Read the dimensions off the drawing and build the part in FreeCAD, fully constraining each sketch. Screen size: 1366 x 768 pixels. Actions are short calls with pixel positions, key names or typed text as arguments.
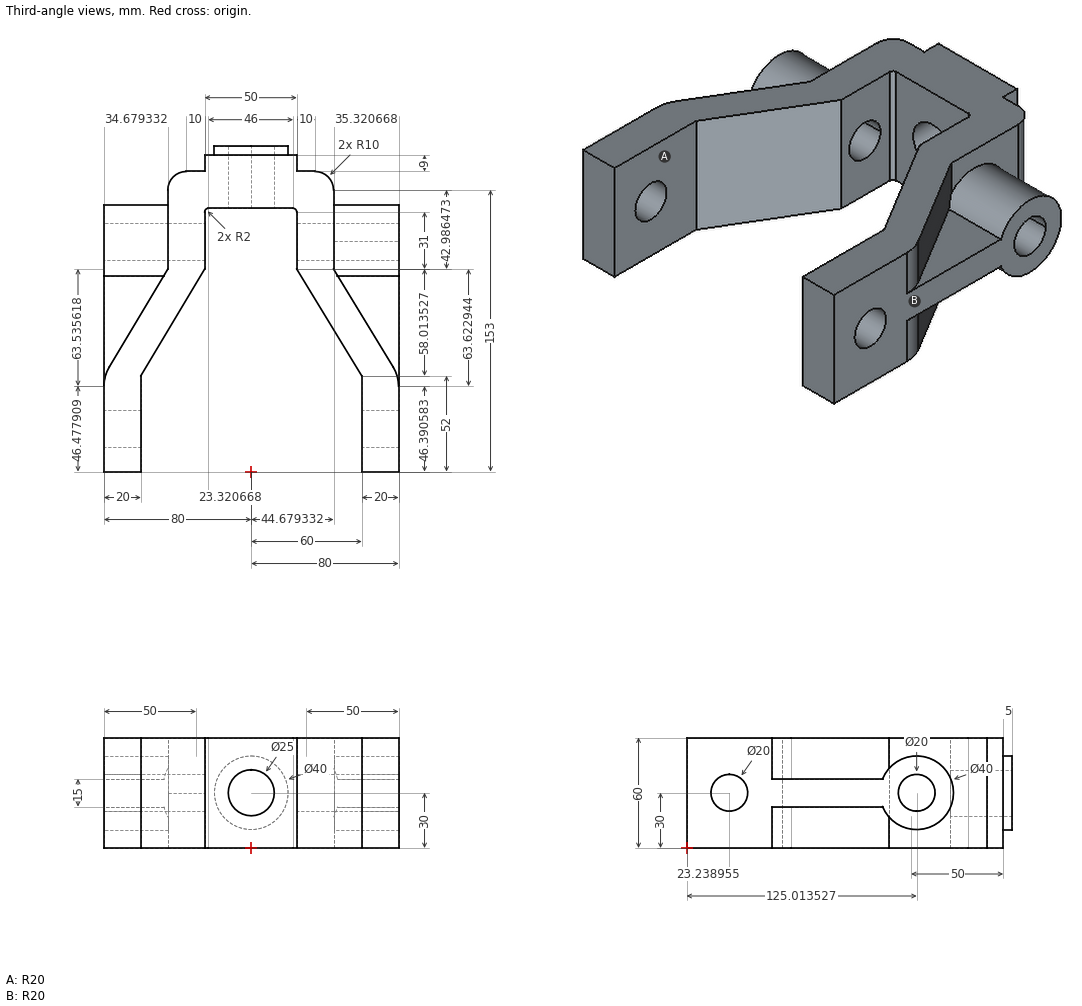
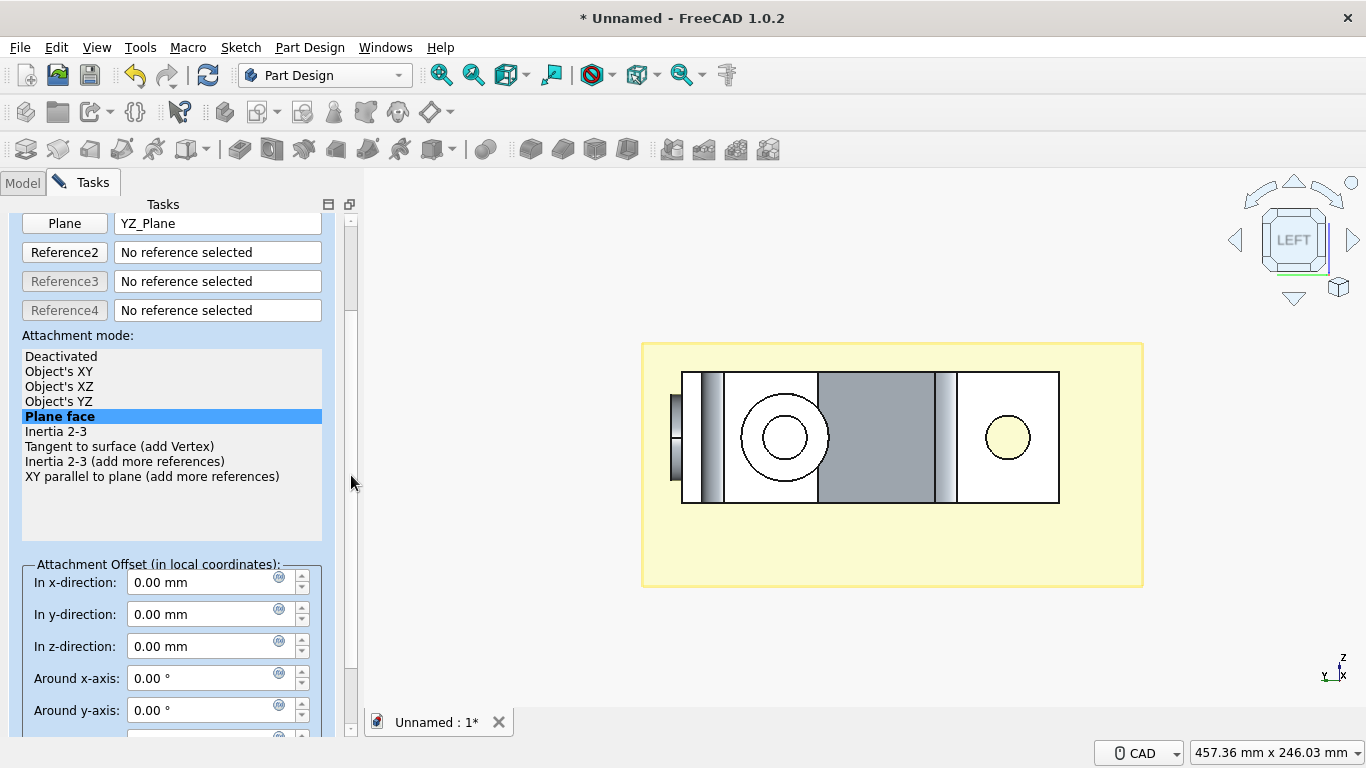
triple_click(210, 646)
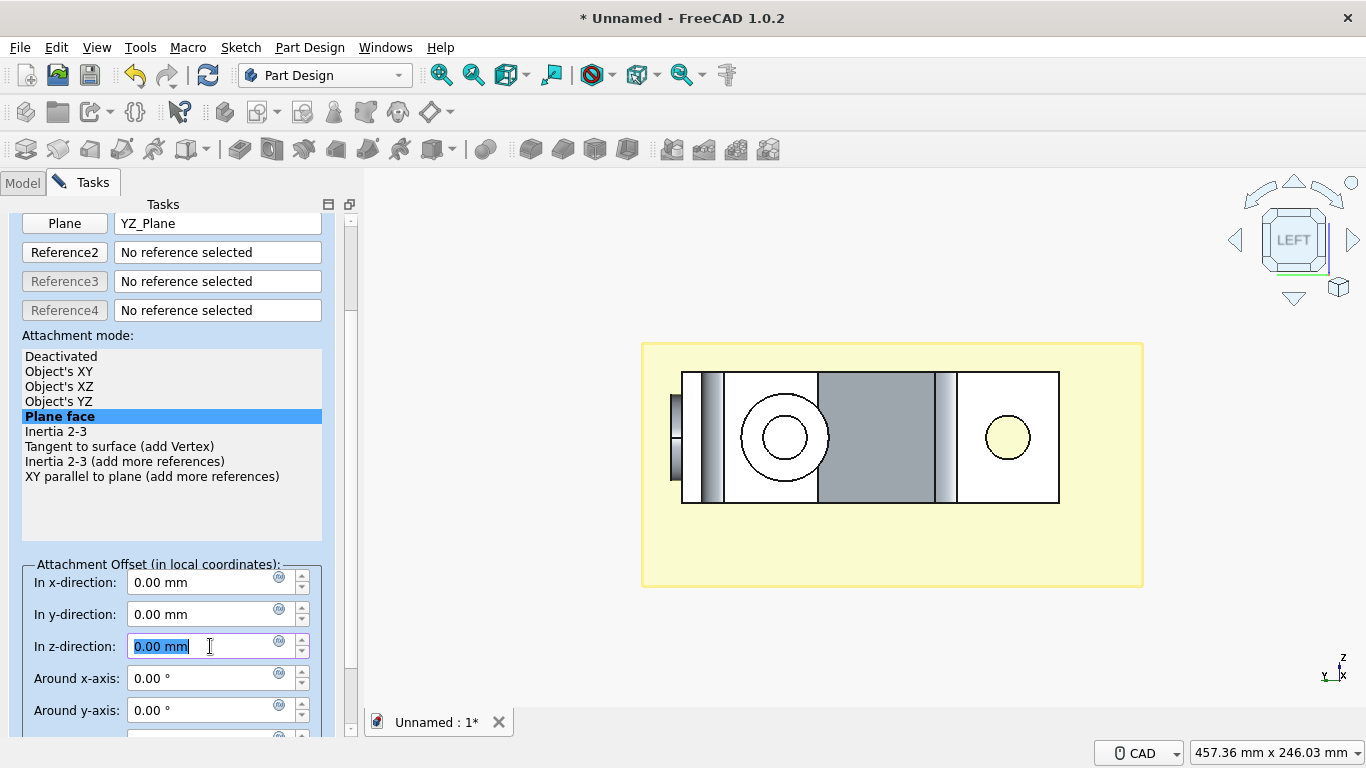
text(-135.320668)
key(Tab)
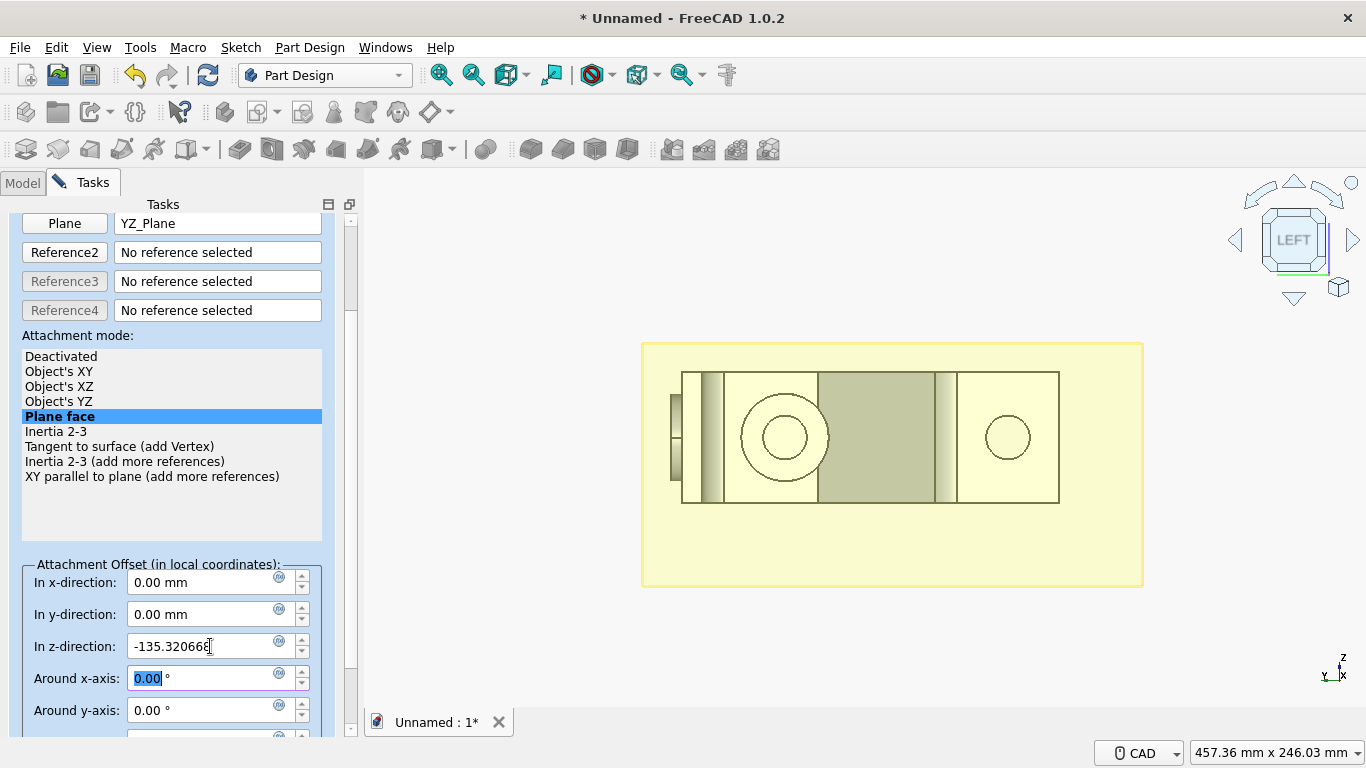
scroll(351, 475, up, 3)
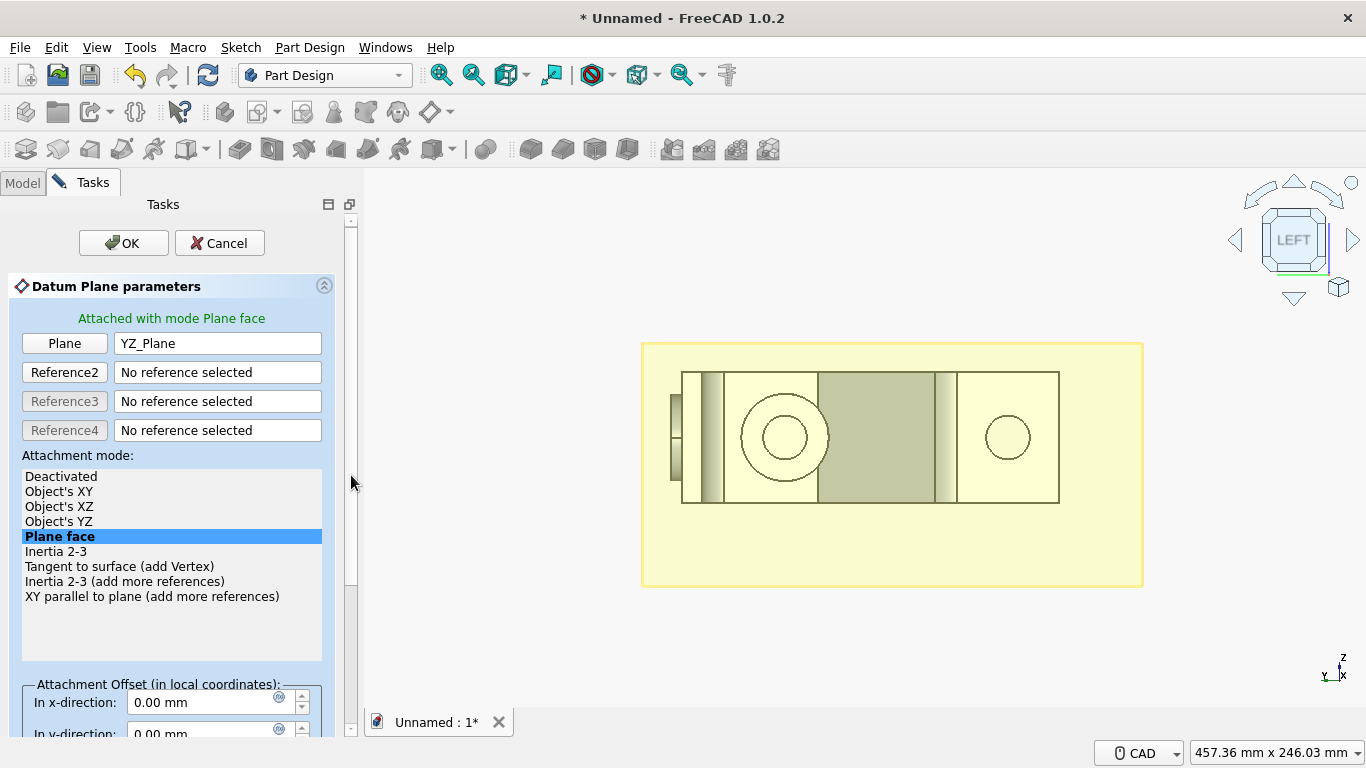
click(124, 243)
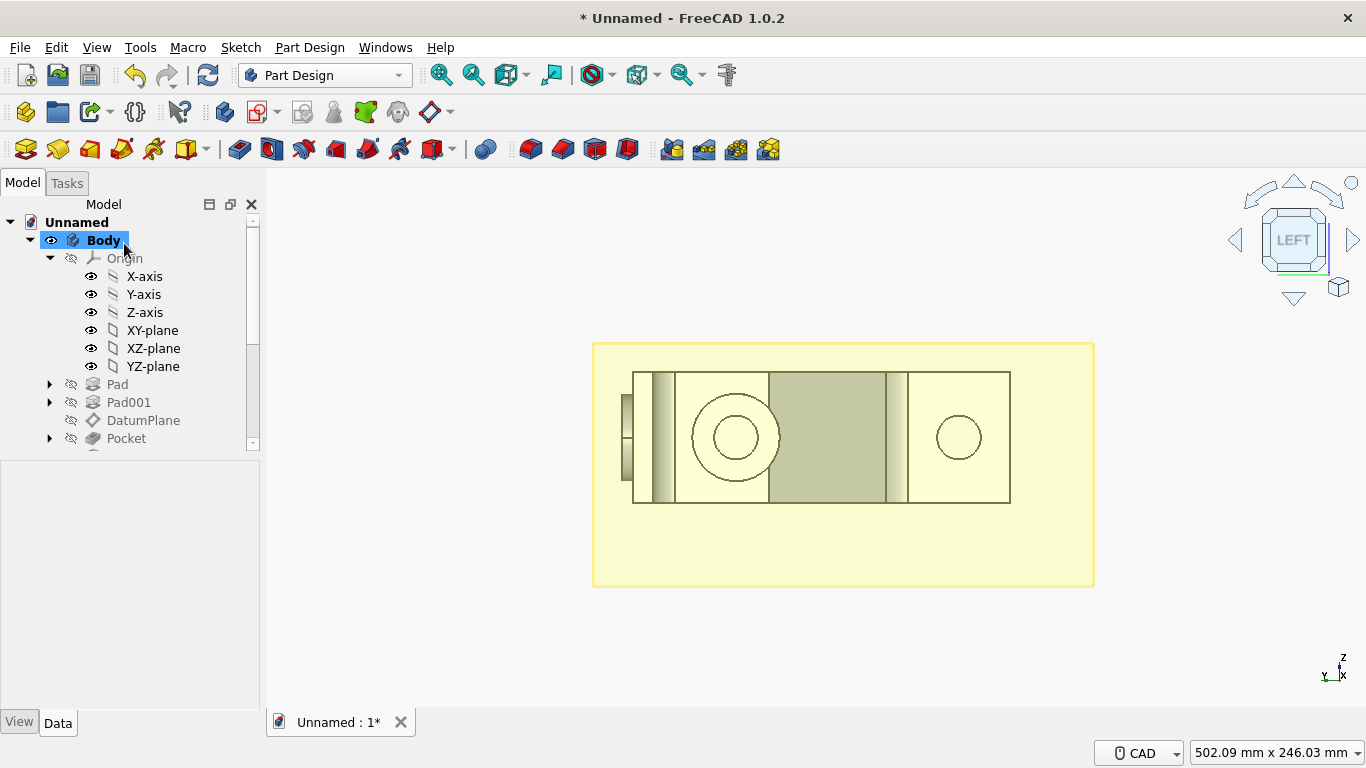
scroll(100, 326, down, 3)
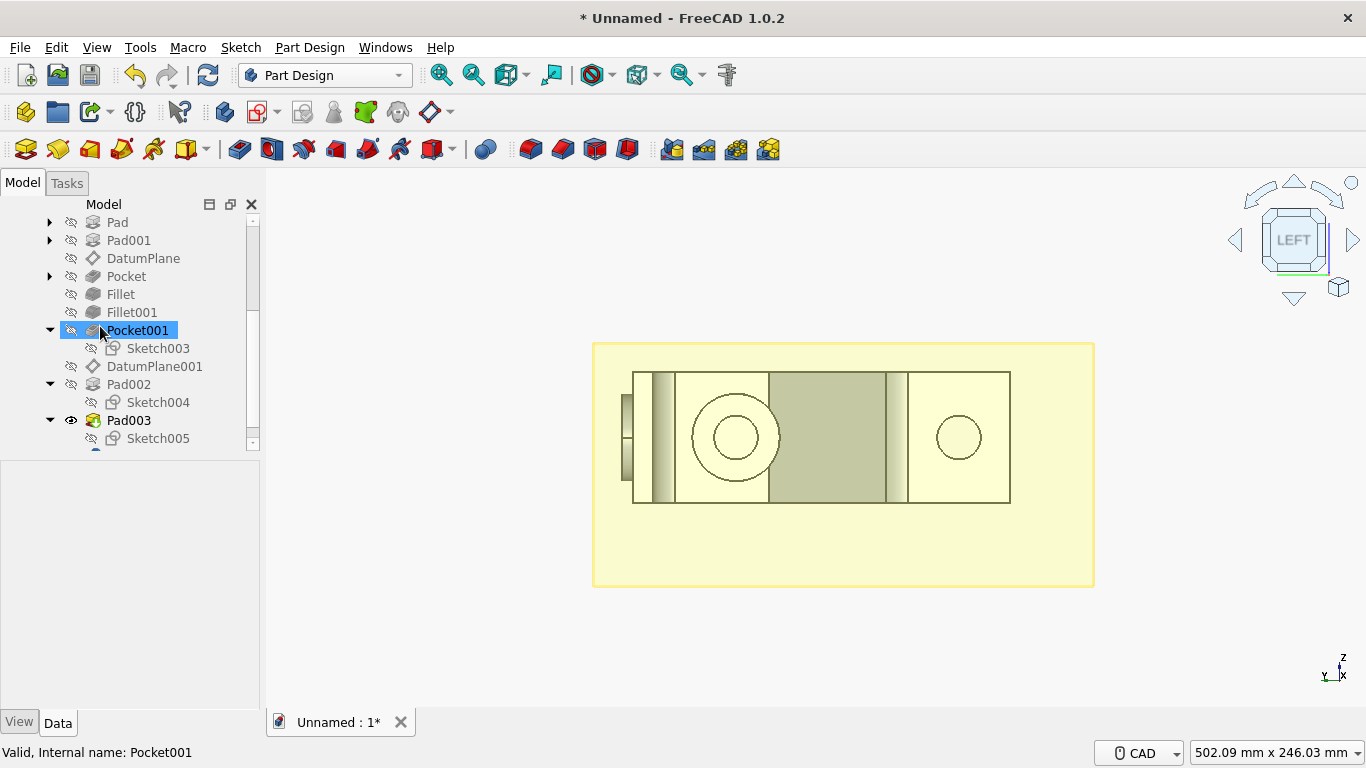
scroll(140, 326, up, 15)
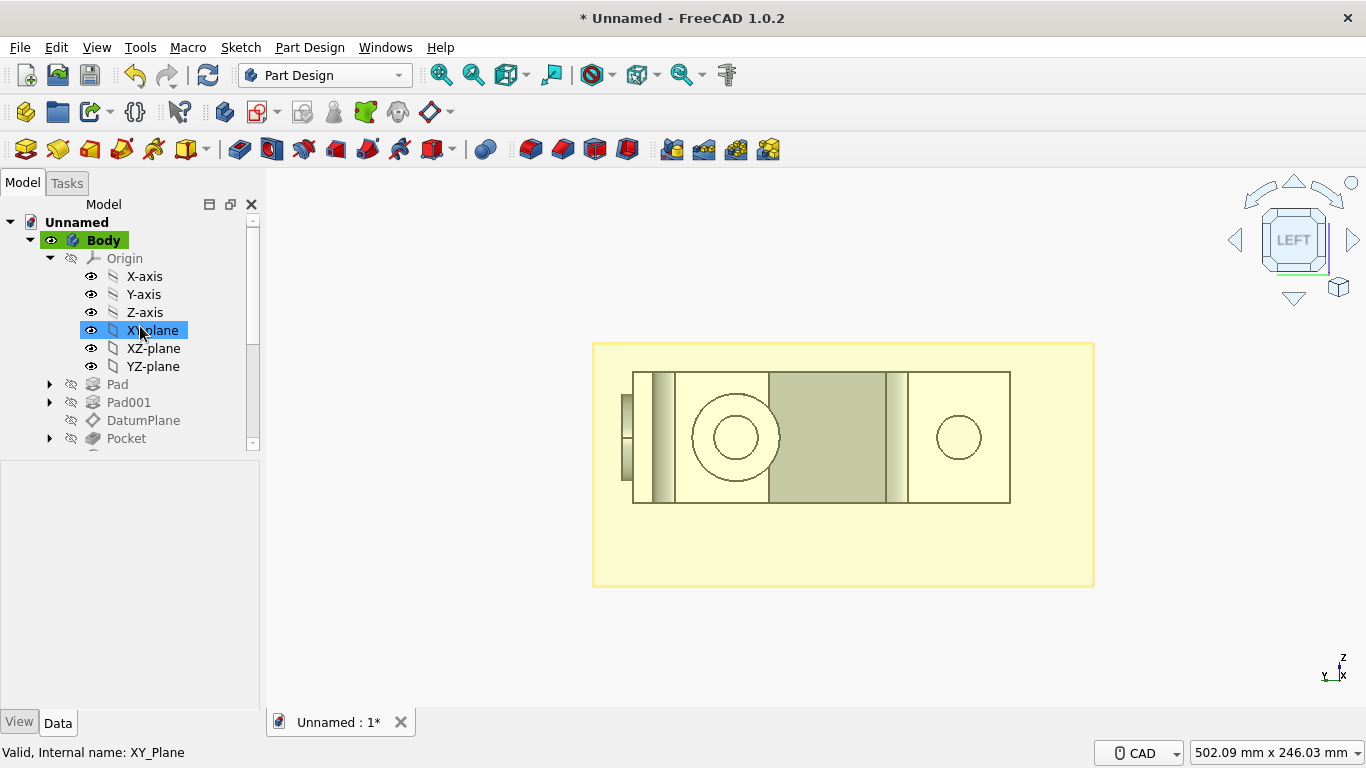
scroll(100, 326, down, 6)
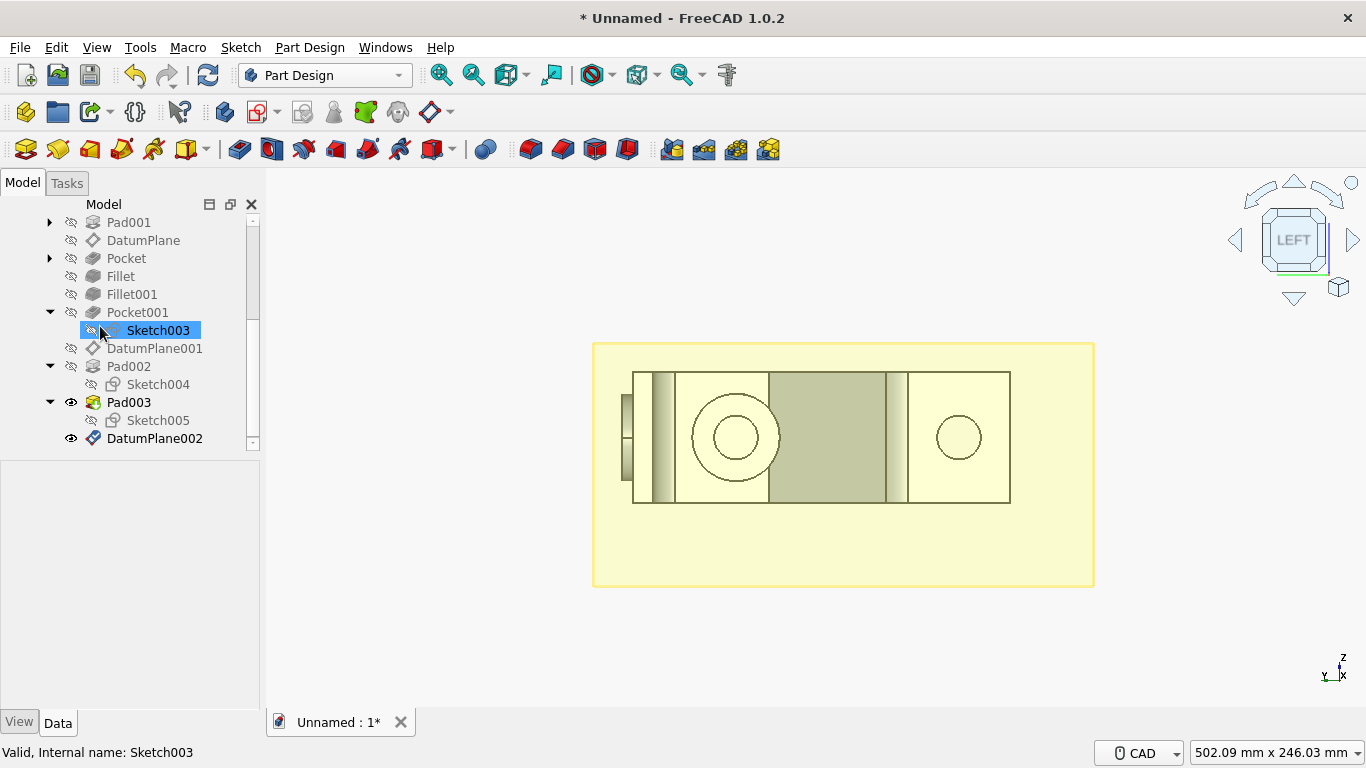
click(116, 438)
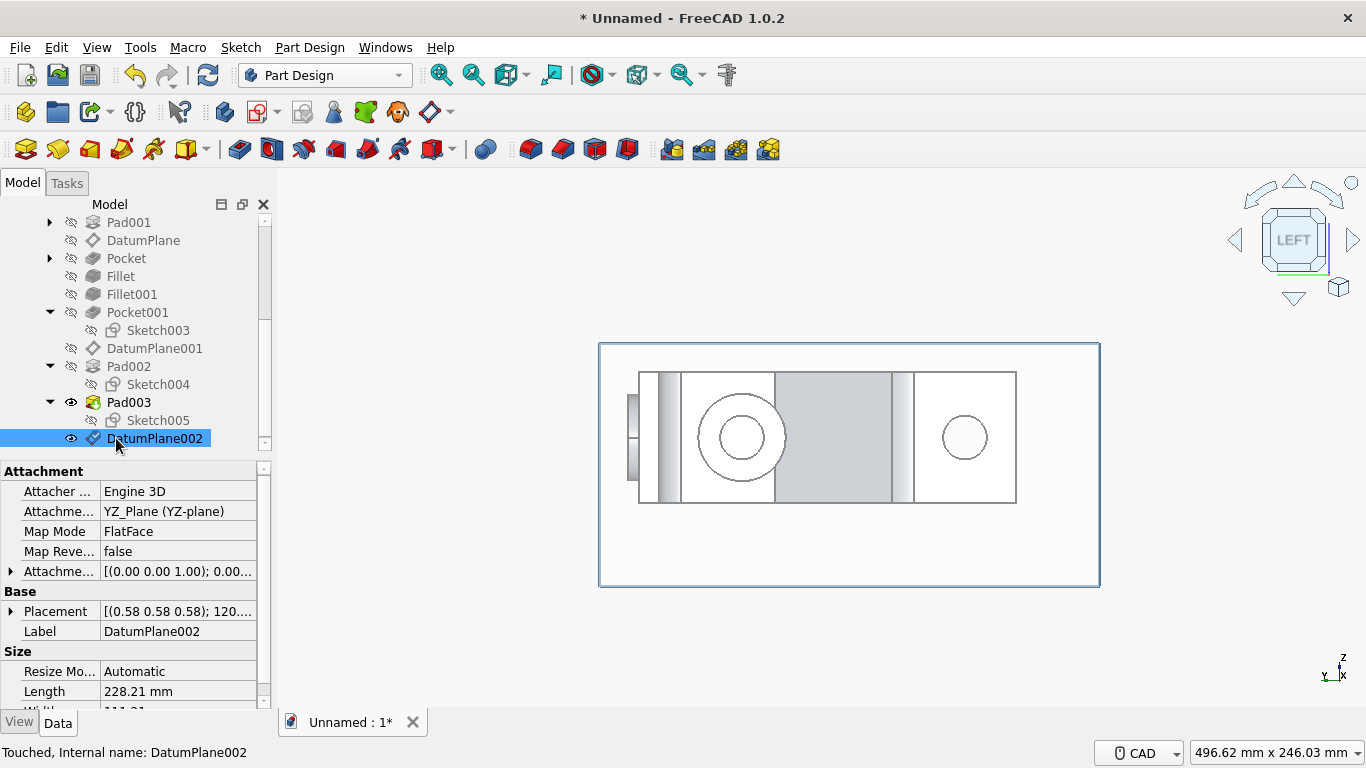
click(258, 112)